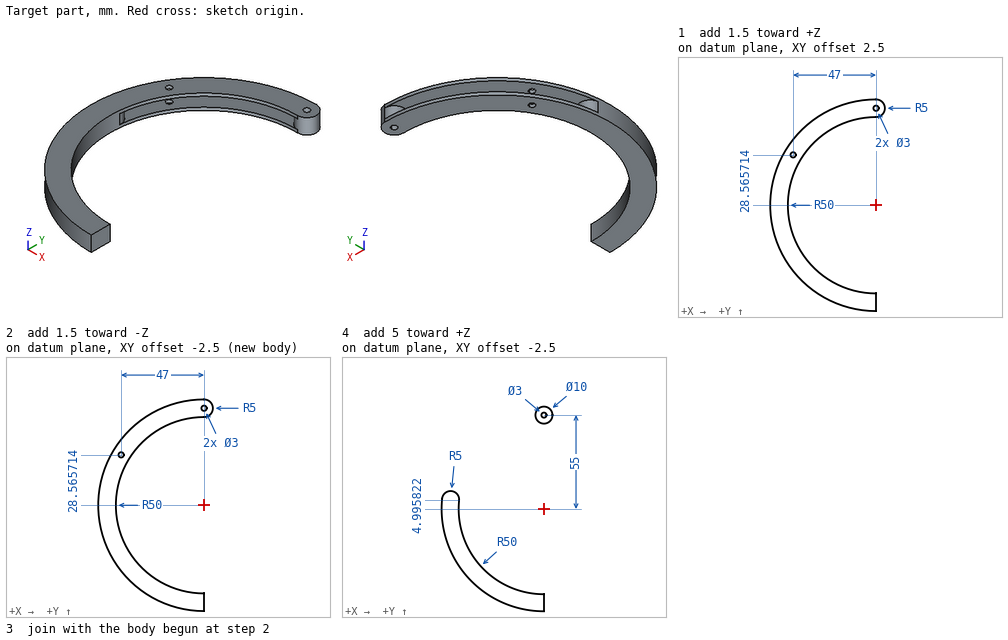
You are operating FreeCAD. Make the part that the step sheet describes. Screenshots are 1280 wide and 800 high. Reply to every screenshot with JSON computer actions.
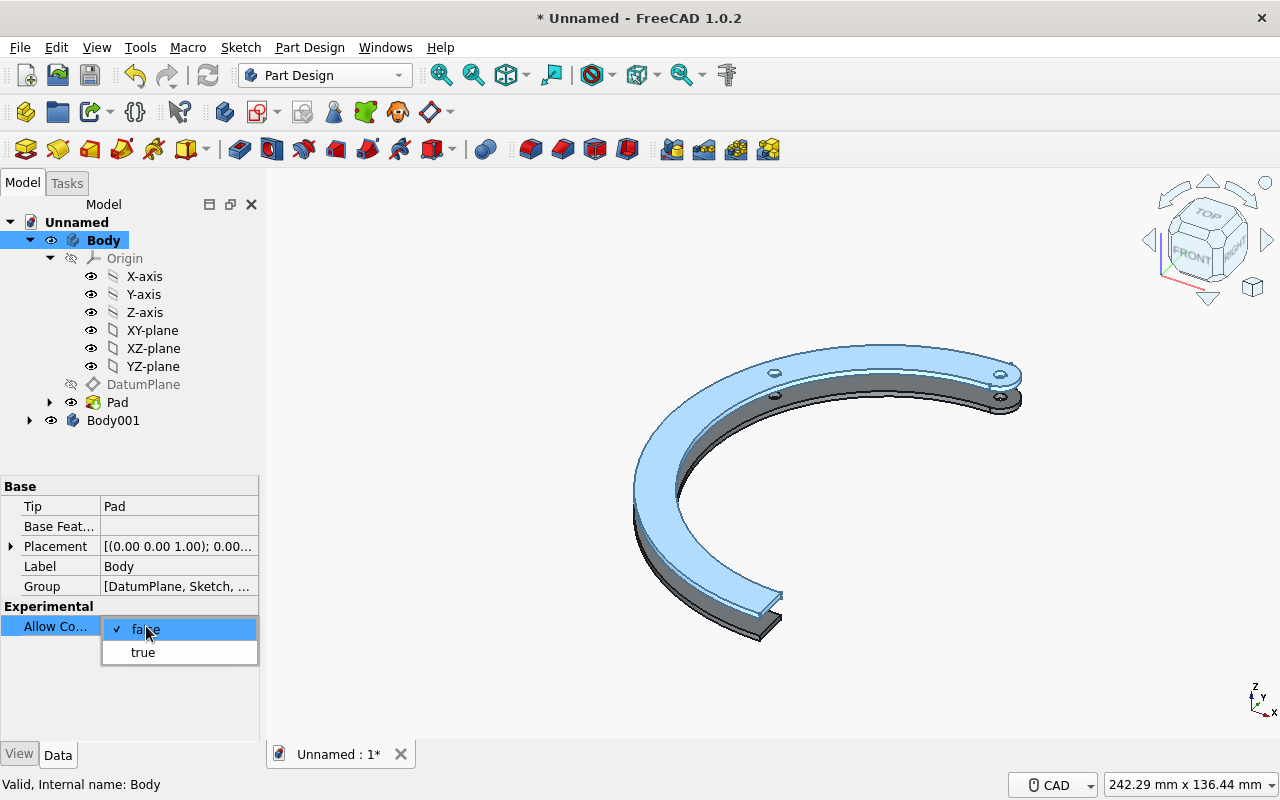
{"action": "left_click", "coordinate": [179, 652]}
{"action": "key", "text": "Return"}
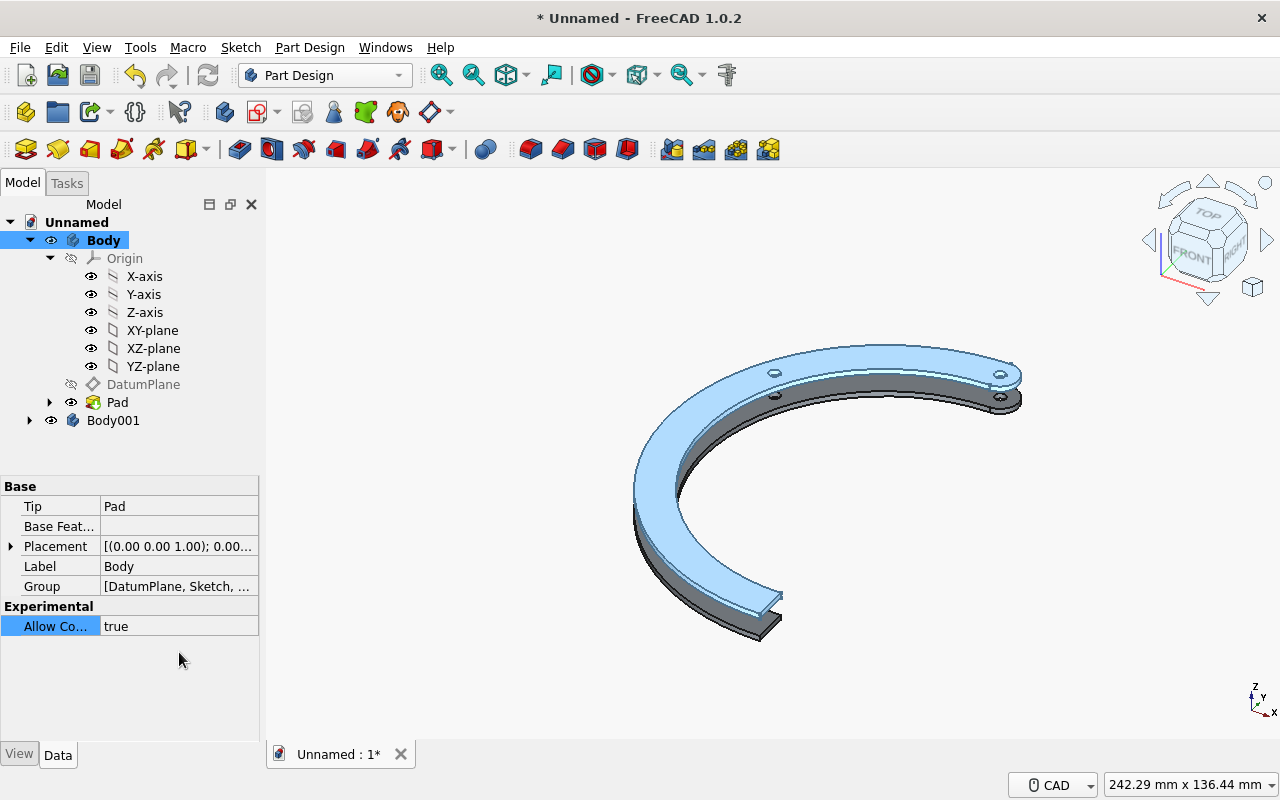
{"action": "left_click", "coordinate": [96, 420]}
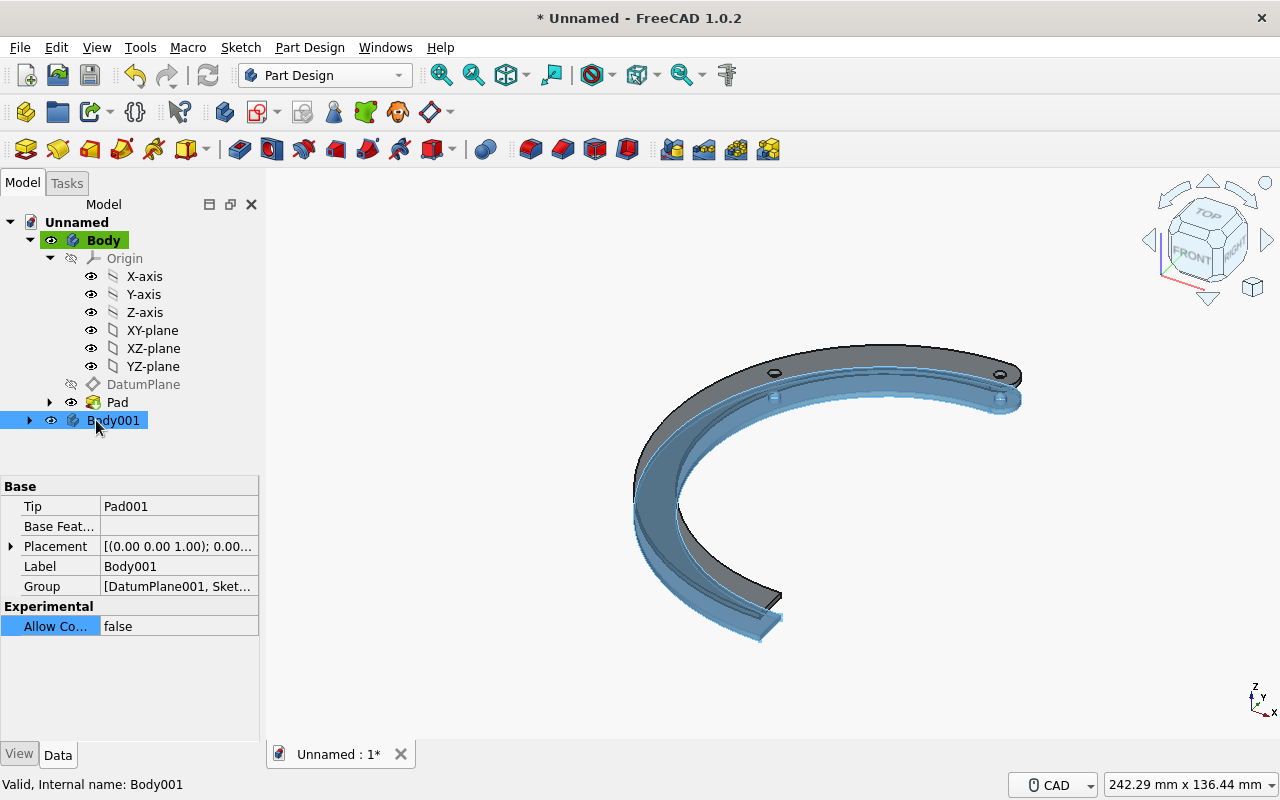
{"action": "left_click", "coordinate": [486, 150]}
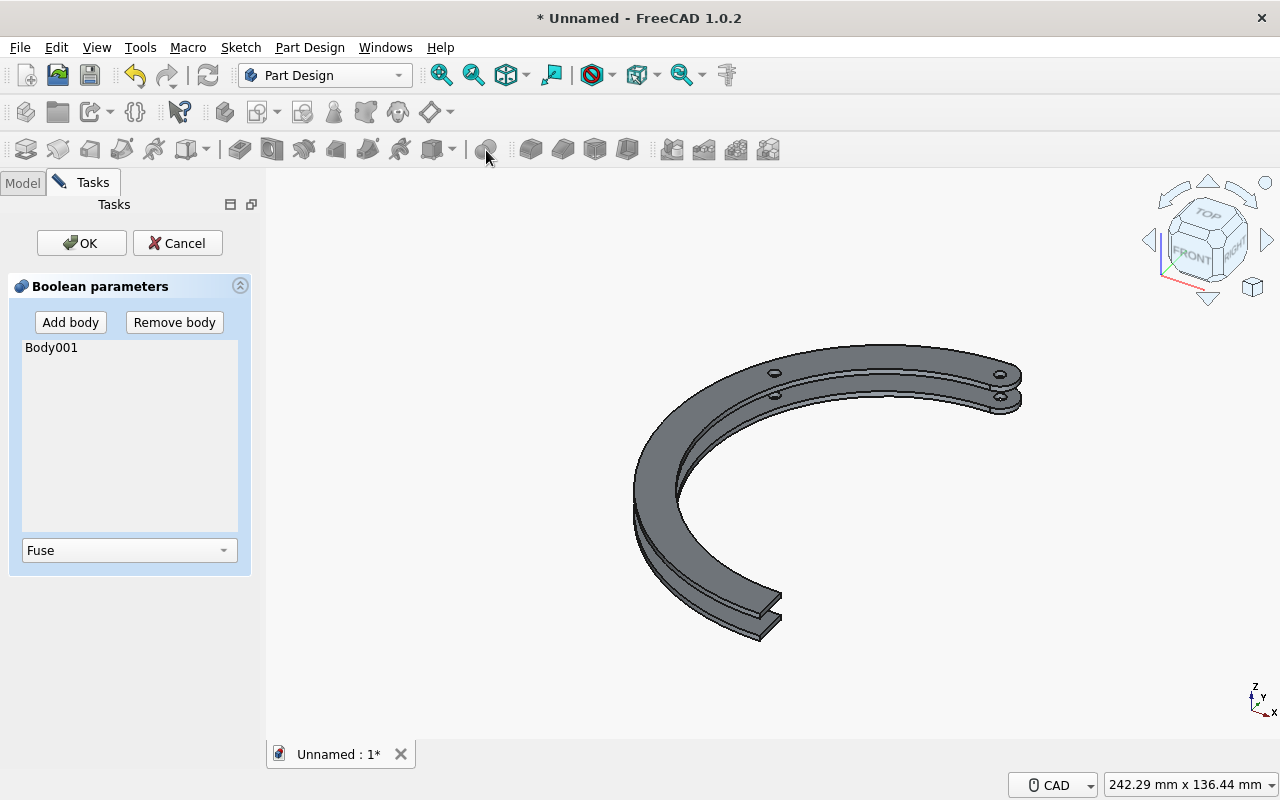
{"action": "left_click", "coordinate": [82, 243]}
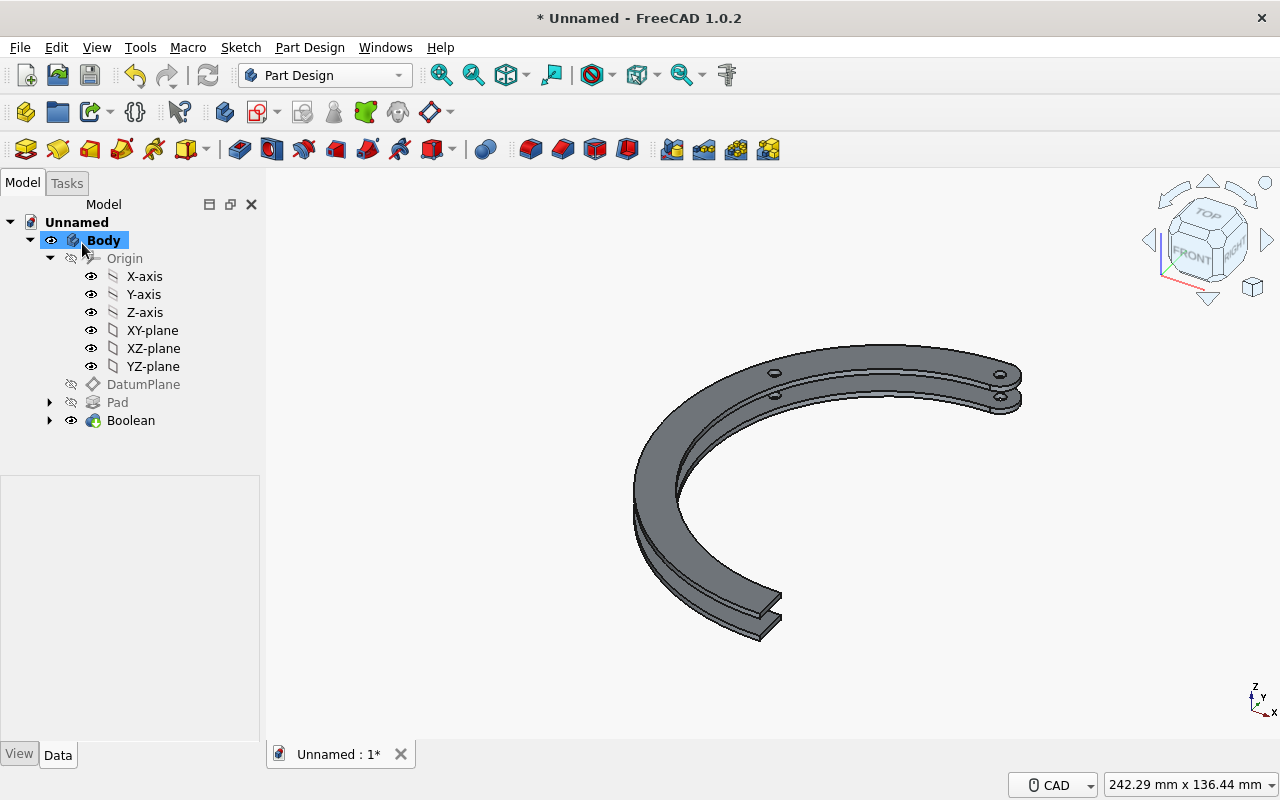
{"action": "left_click", "coordinate": [136, 330]}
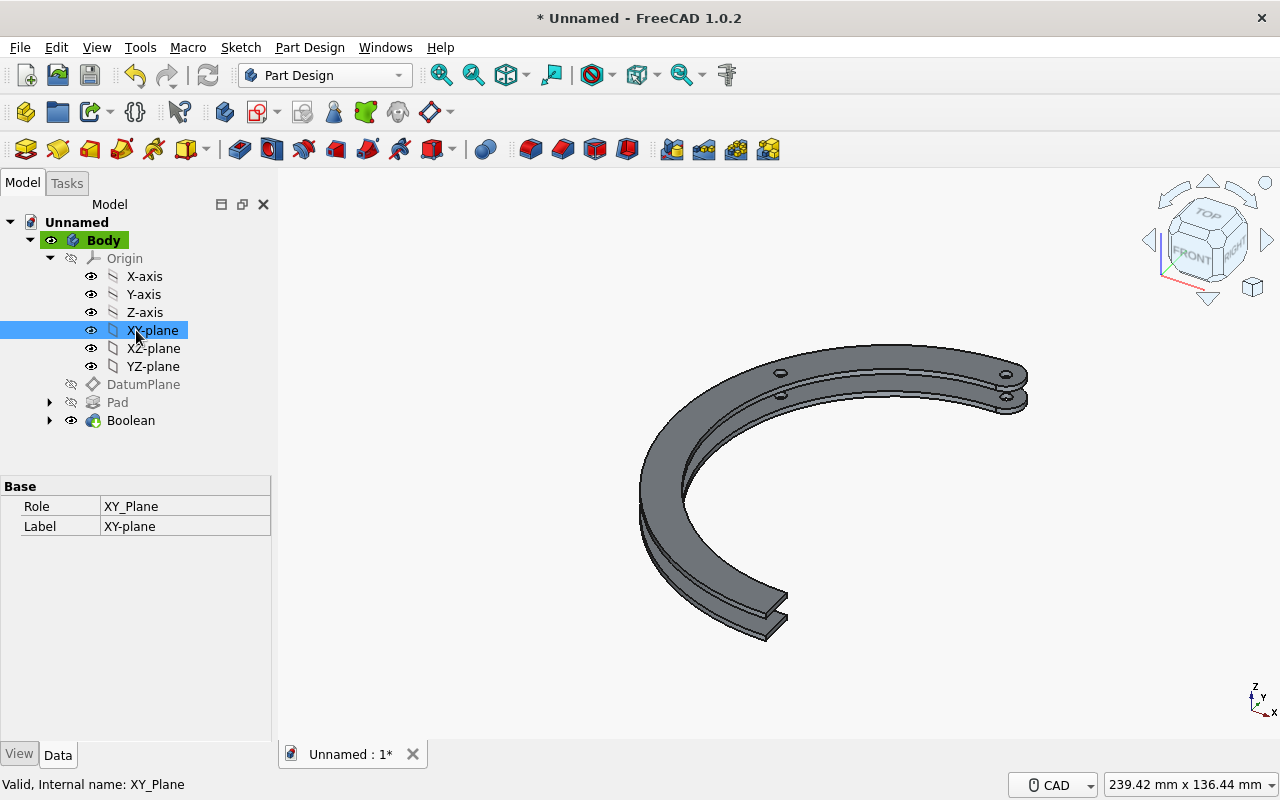
{"action": "left_click", "coordinate": [430, 112]}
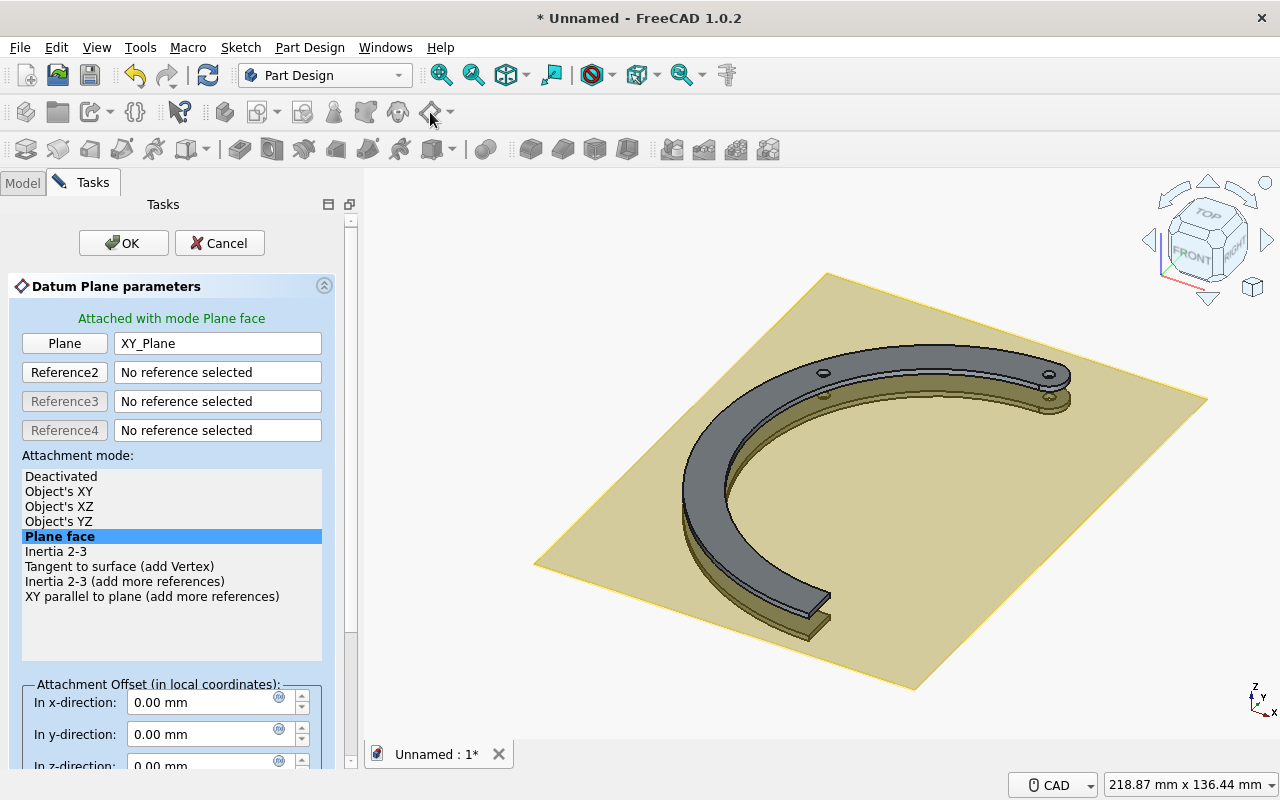
{"action": "scroll", "coordinate": [351, 491], "scroll_direction": "down", "scroll_amount": 2}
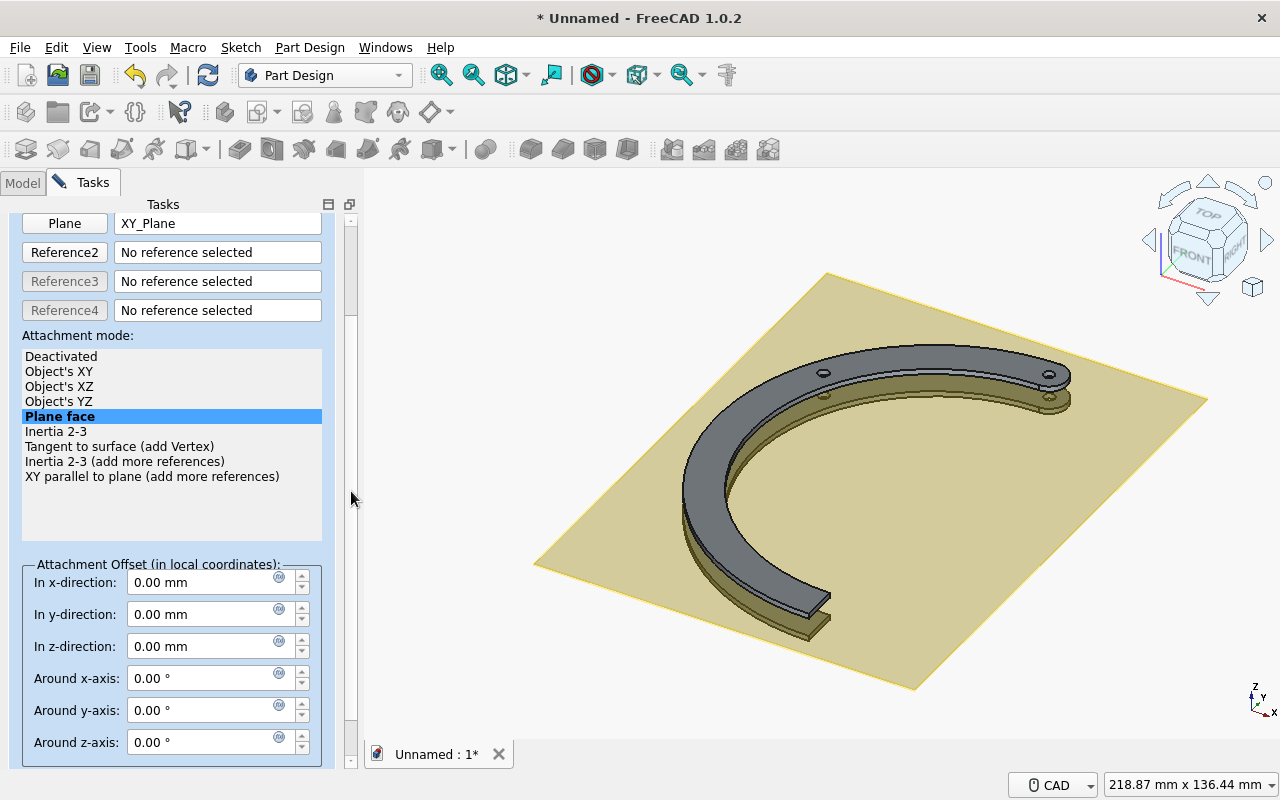
{"action": "triple_click", "coordinate": [210, 646]}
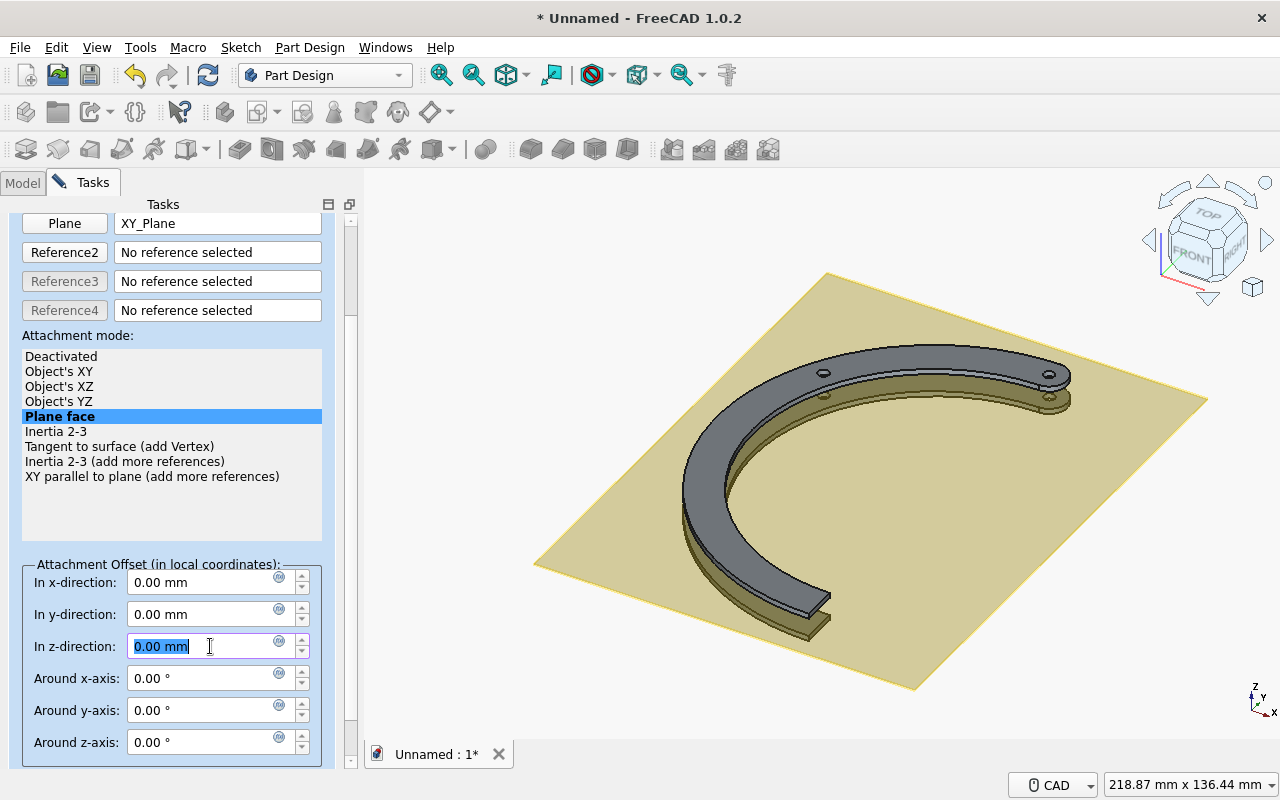
{"action": "type", "text": "-2.5"}
{"action": "key", "text": "Tab"}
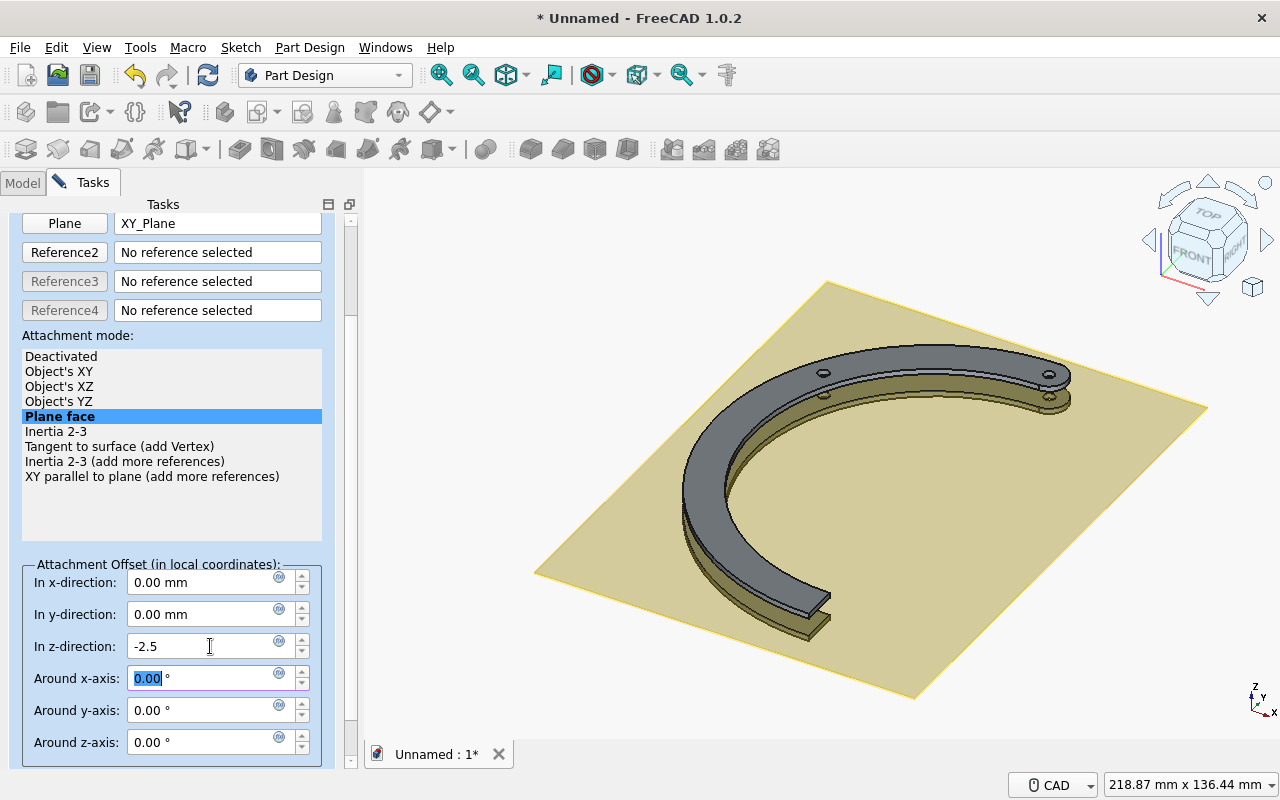
{"action": "scroll", "coordinate": [351, 491], "scroll_direction": "up", "scroll_amount": 3}